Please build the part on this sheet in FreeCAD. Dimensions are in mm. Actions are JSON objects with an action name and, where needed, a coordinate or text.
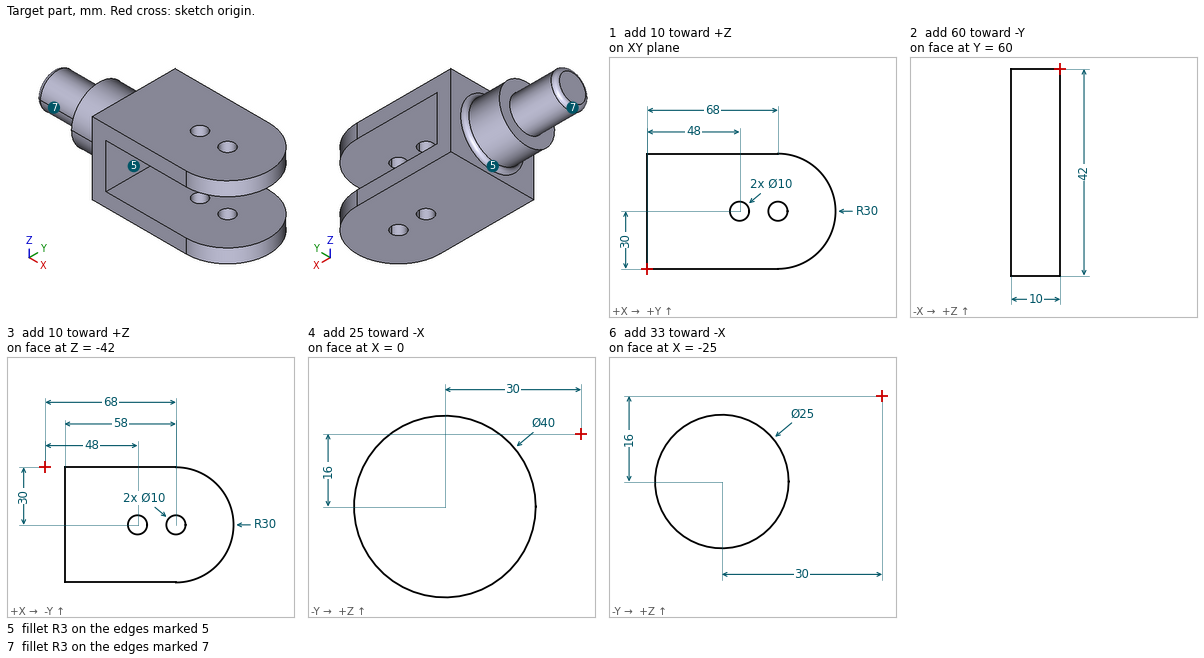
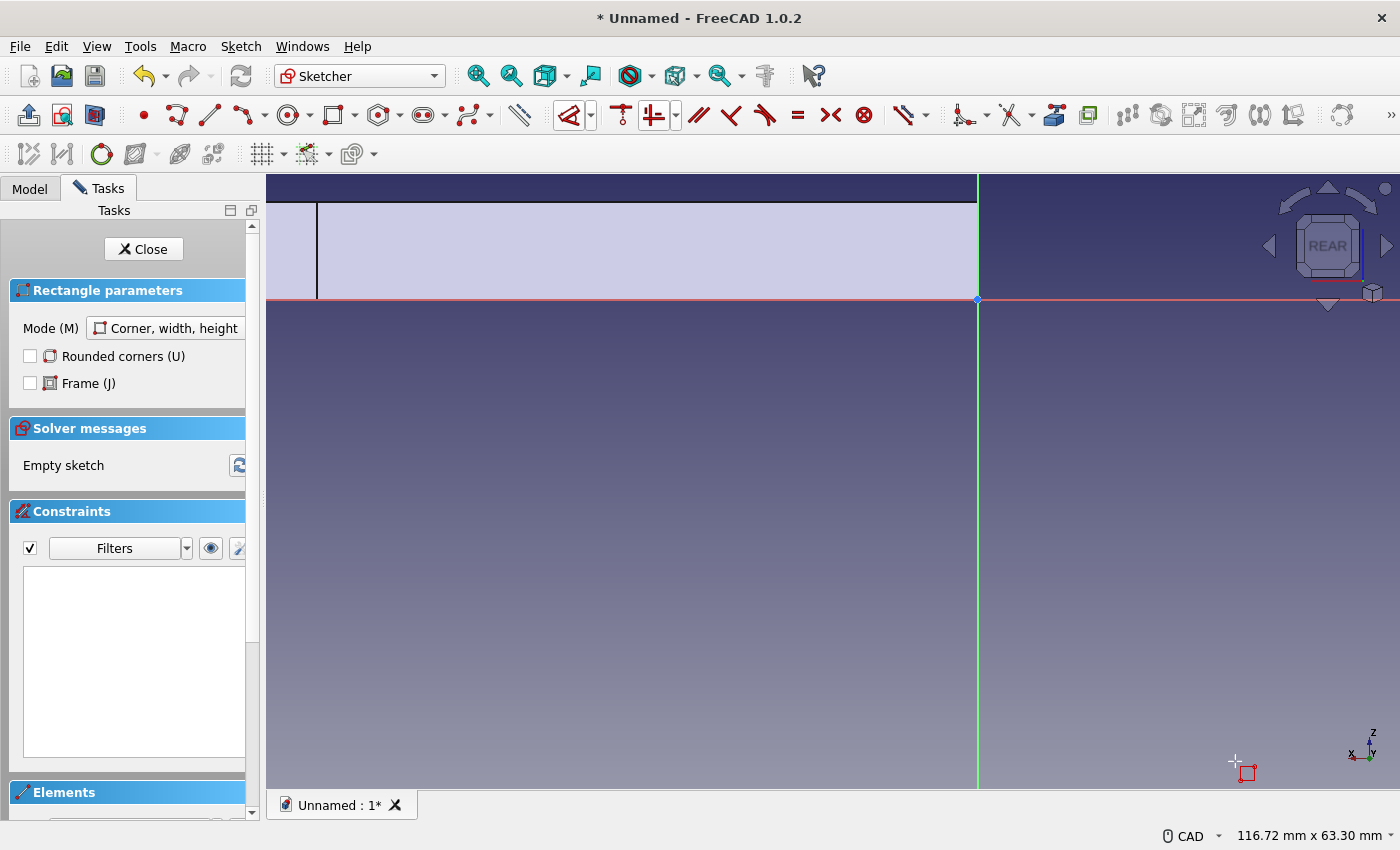
{"action": "left_click", "coordinate": [978, 300]}
{"action": "mouse_move", "coordinate": [881, 708]}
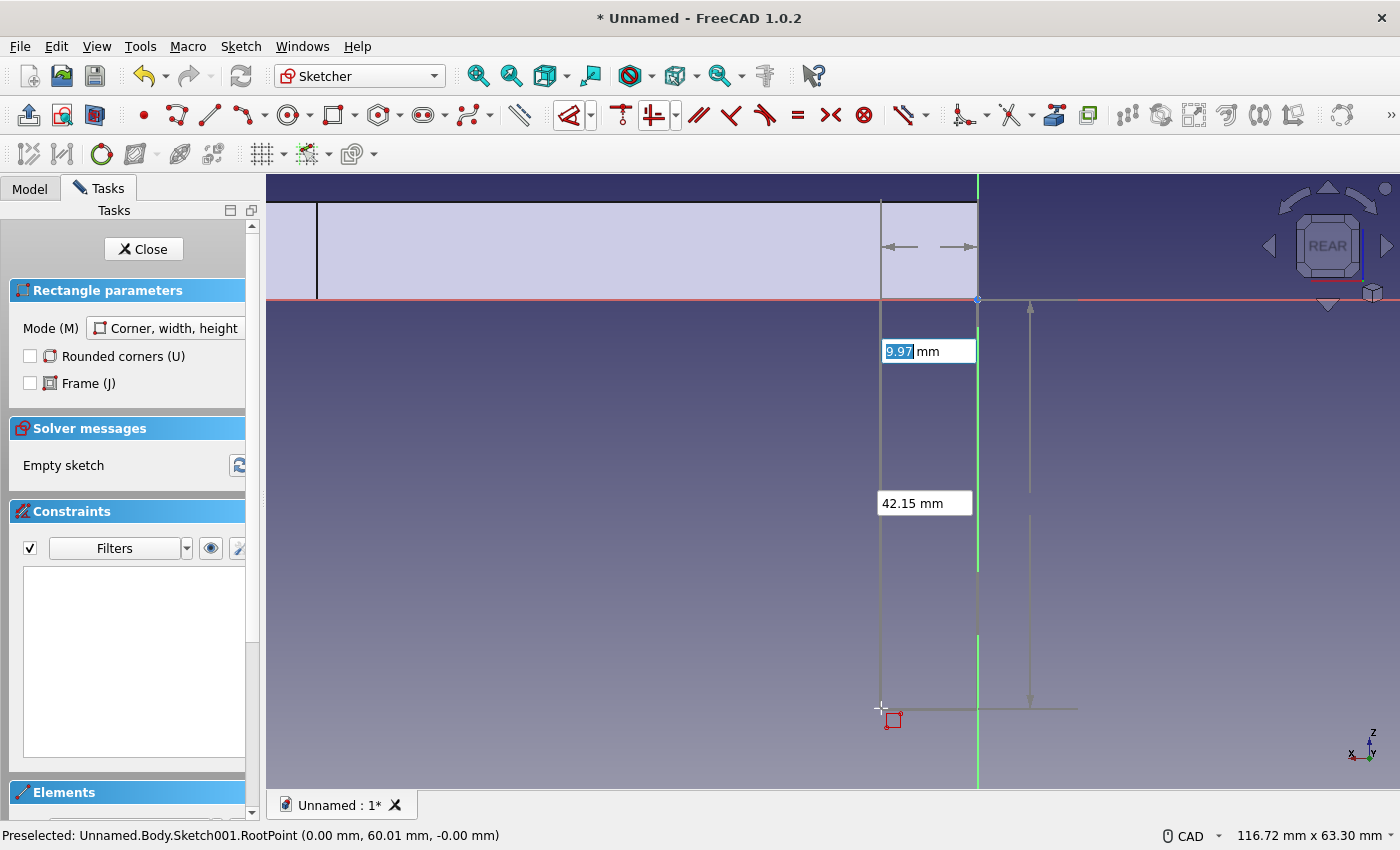
{"action": "type", "text": "10"}
{"action": "key", "text": "Tab"}
{"action": "type", "text": "42"}
{"action": "key", "text": "Return"}
{"action": "key", "text": "Escape"}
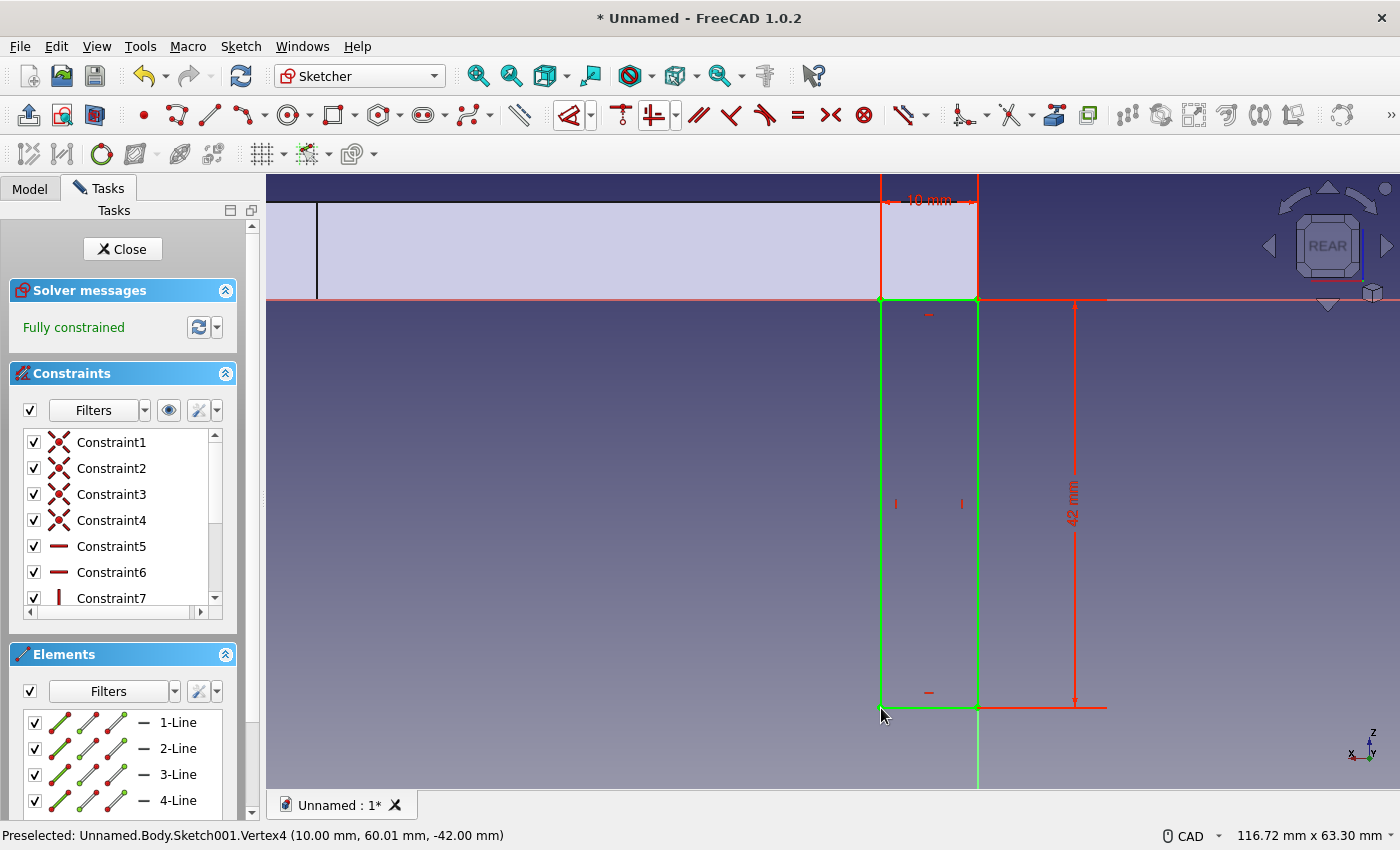
{"action": "left_click", "coordinate": [123, 249]}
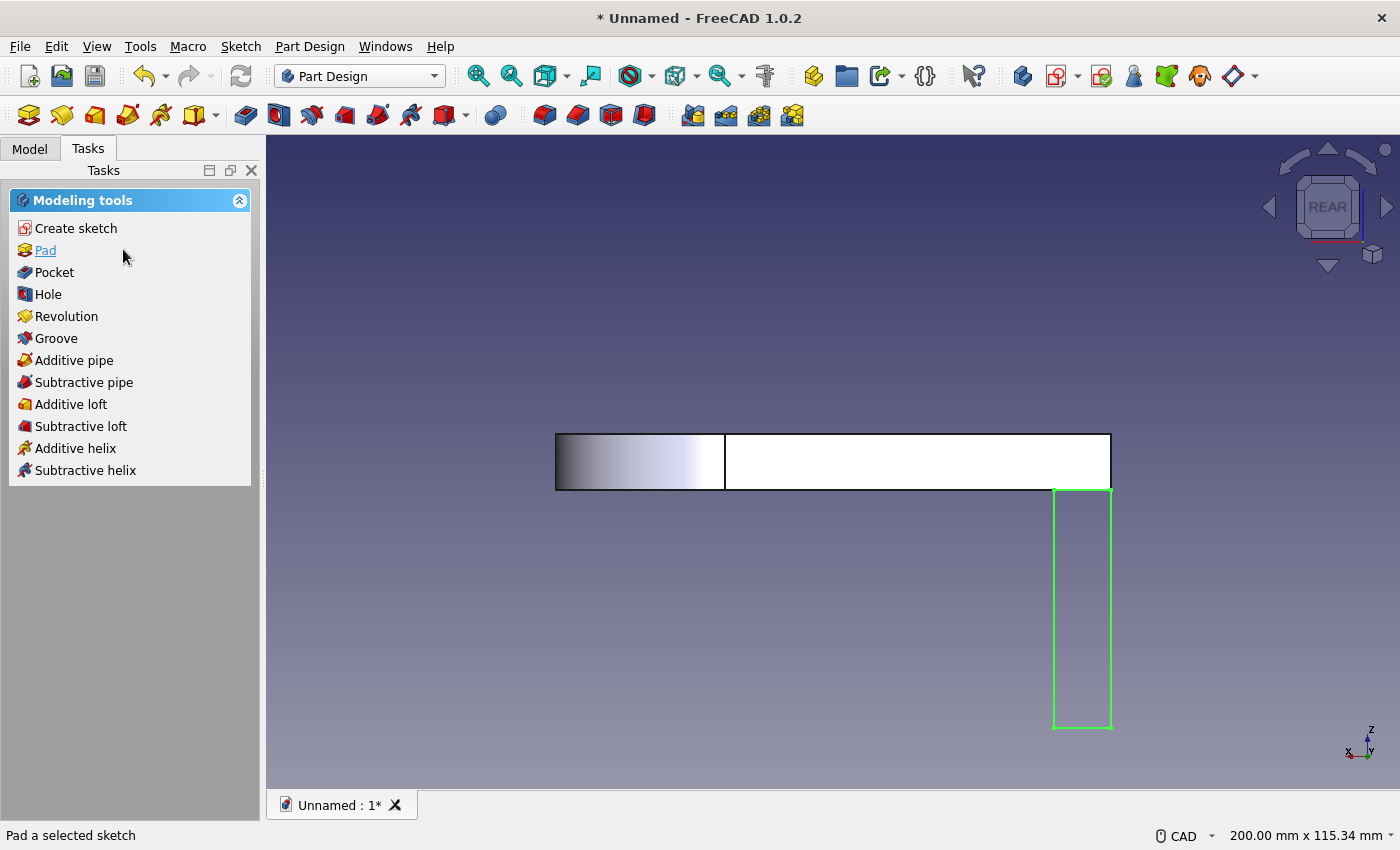
{"action": "left_click", "coordinate": [29, 116]}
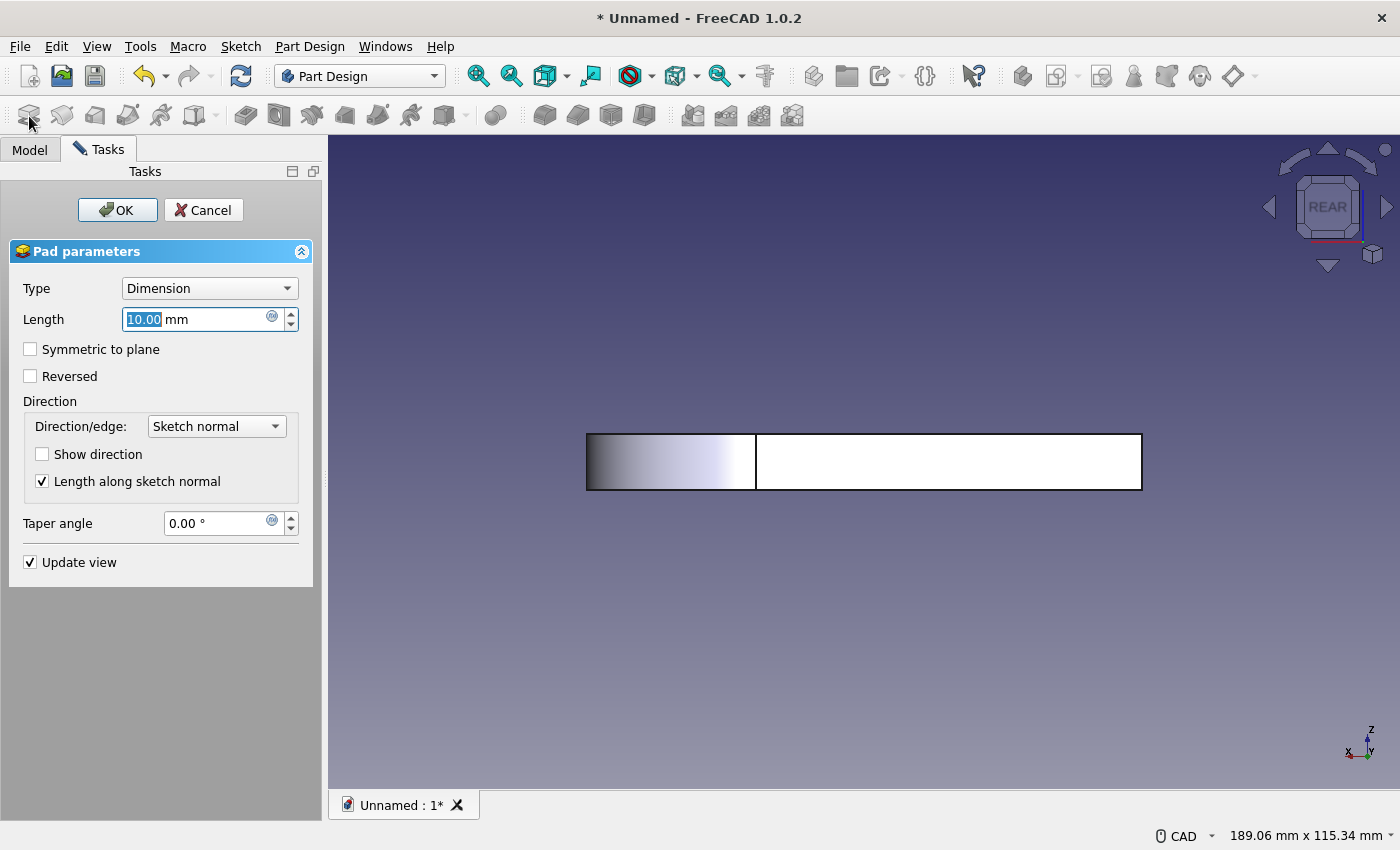
{"action": "type", "text": "60"}
{"action": "key", "text": "Tab"}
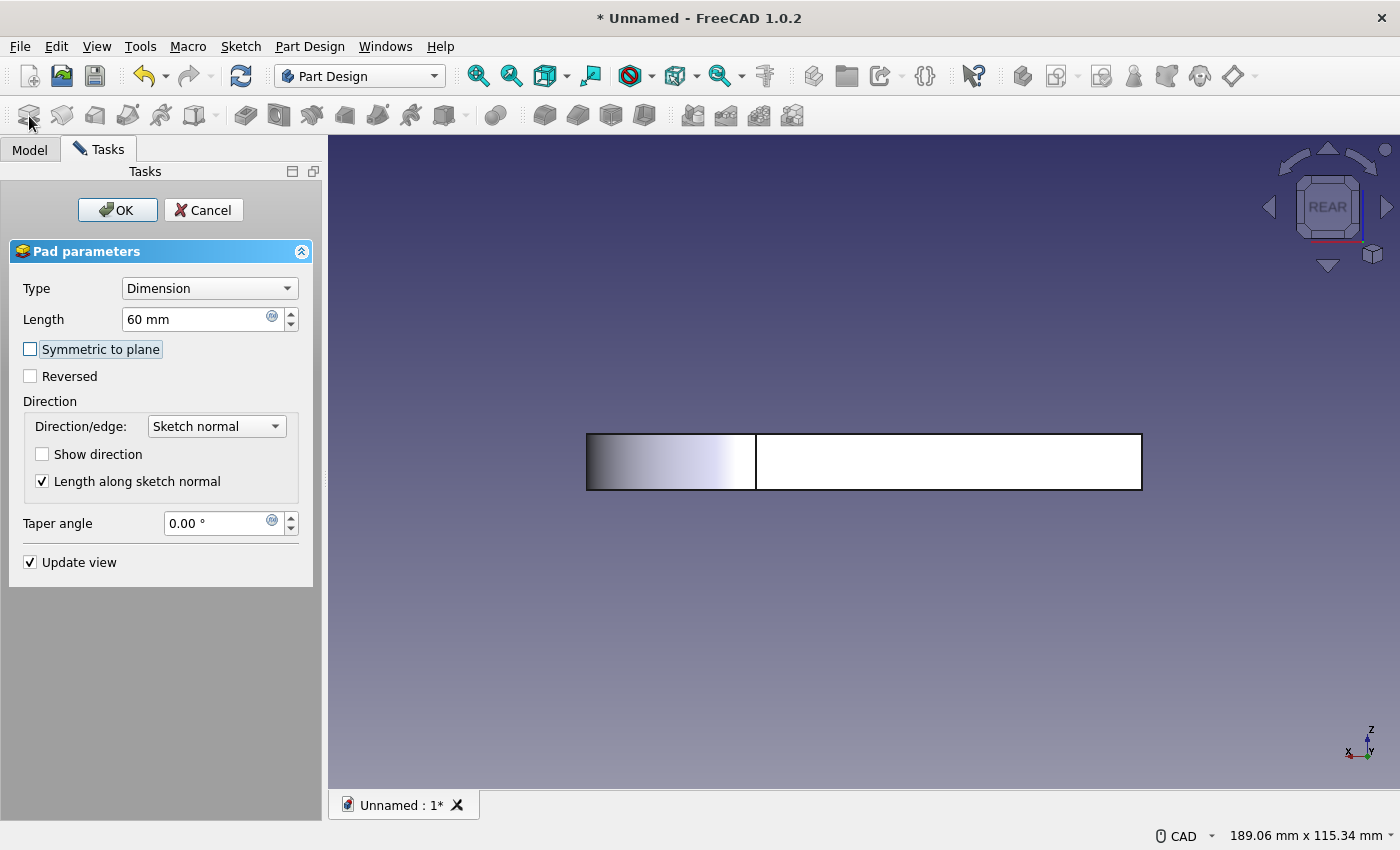
{"action": "left_click", "coordinate": [31, 376]}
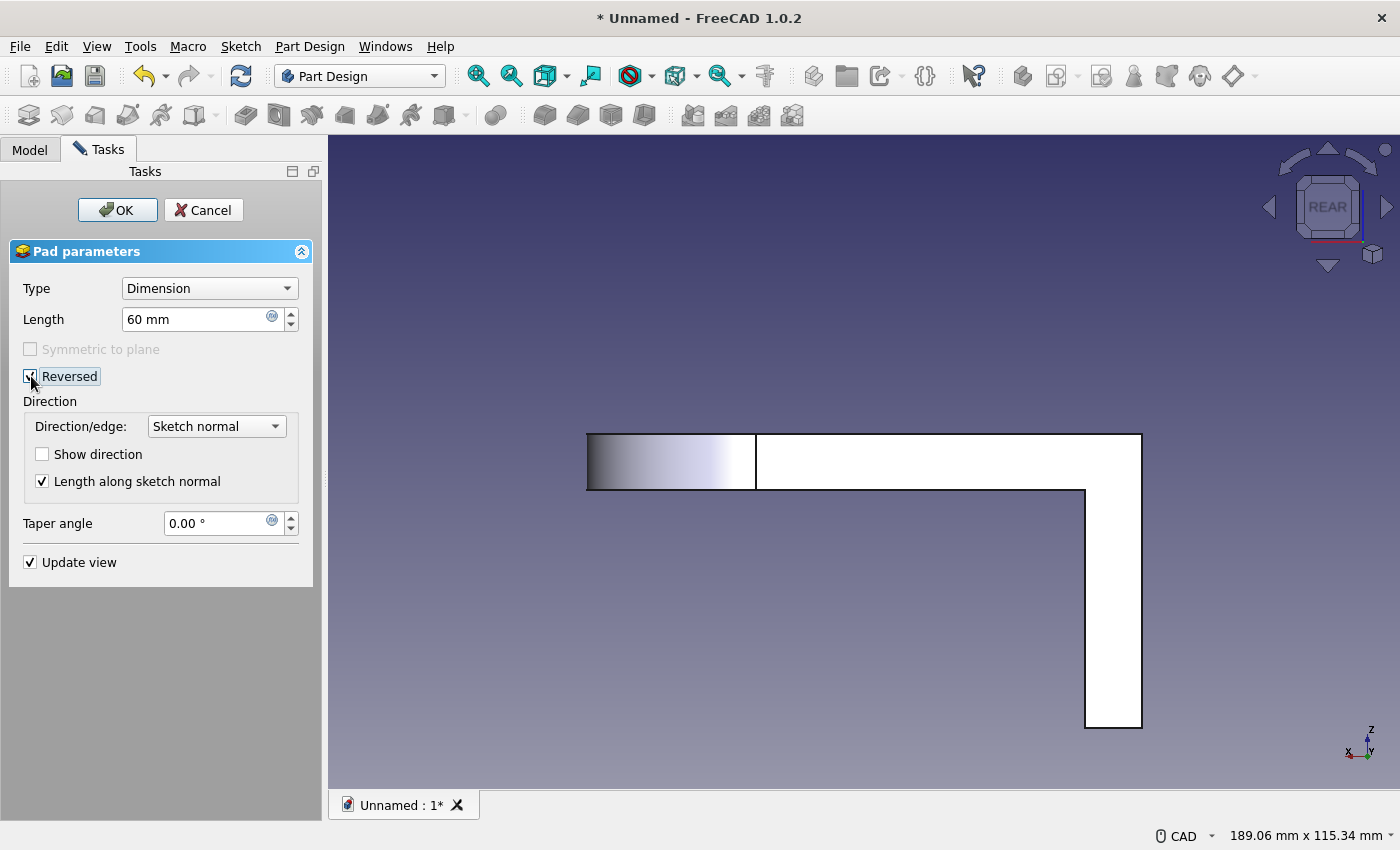
{"action": "left_click", "coordinate": [118, 210]}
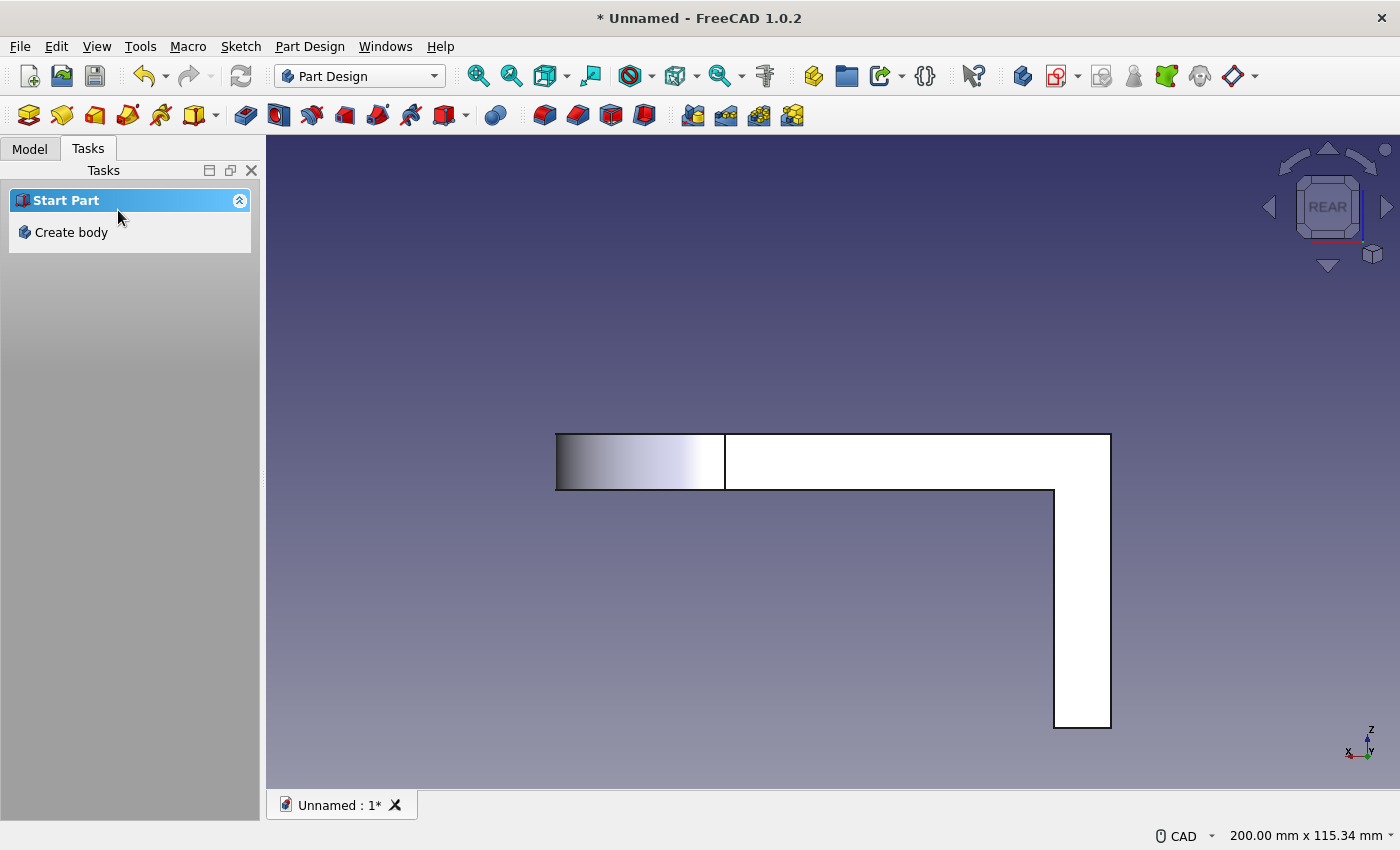
{"action": "key", "text": "5"}